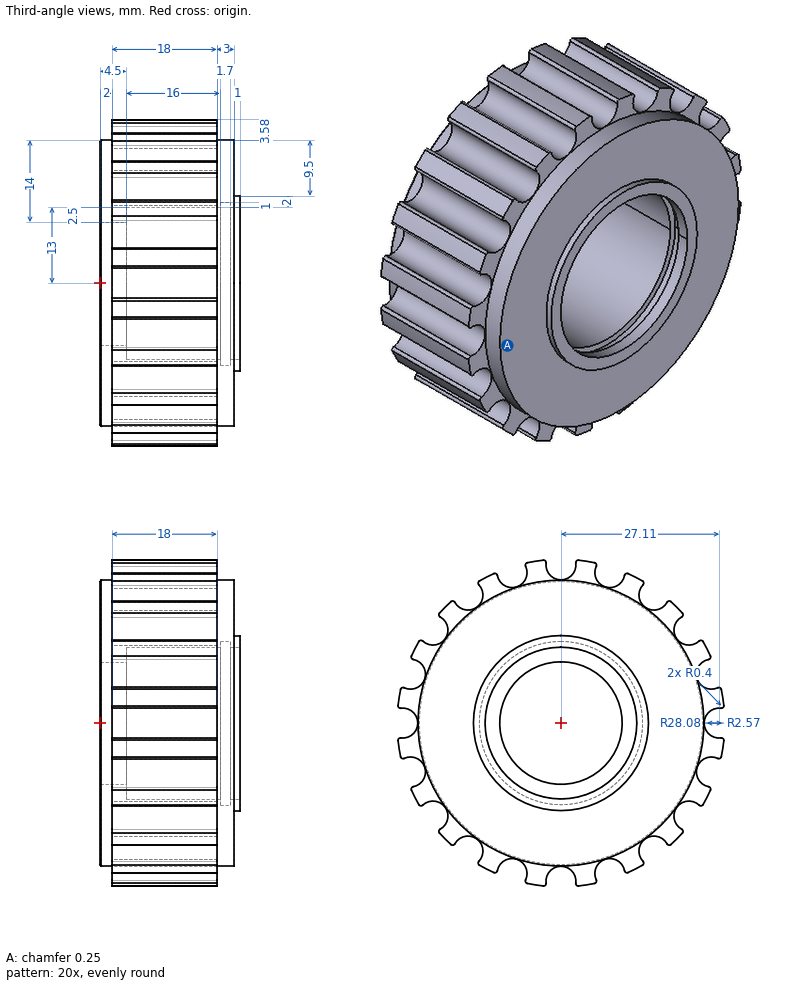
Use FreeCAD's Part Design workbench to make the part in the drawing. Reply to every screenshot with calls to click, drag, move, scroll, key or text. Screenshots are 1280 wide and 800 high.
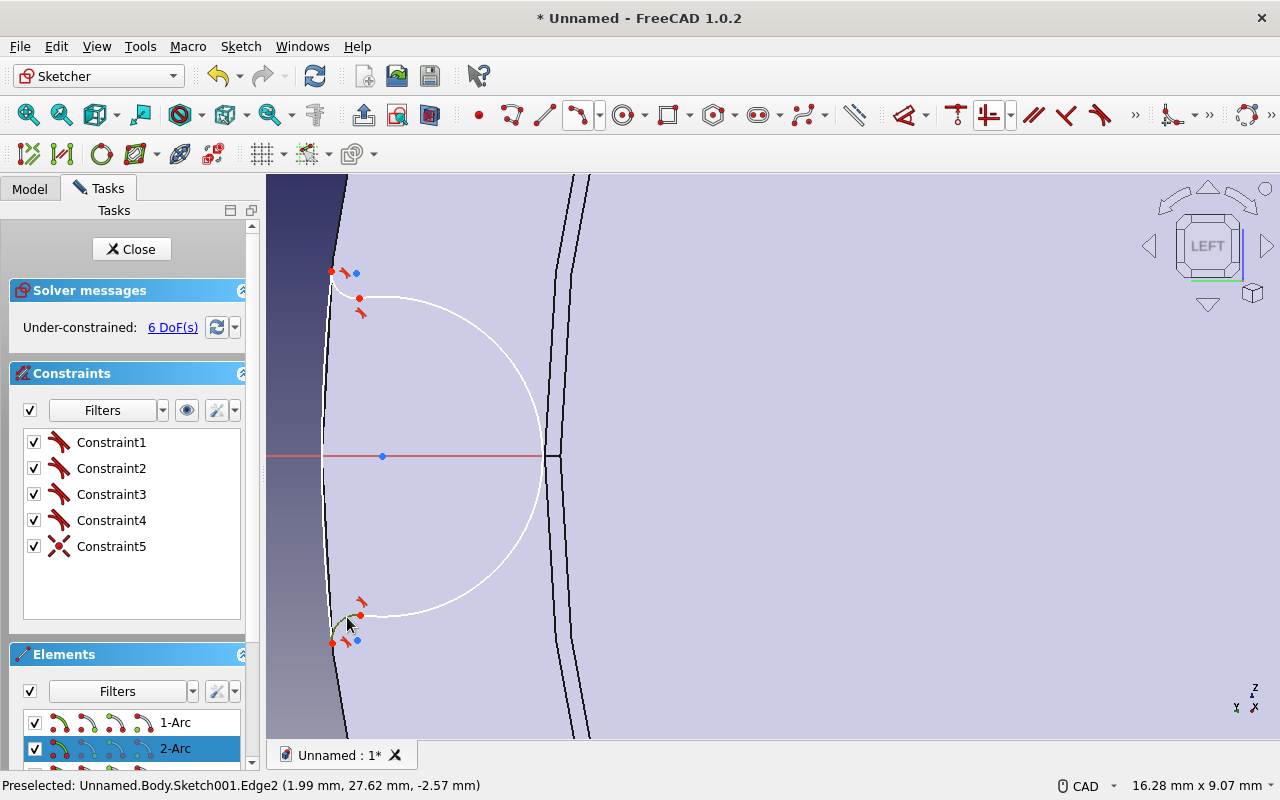
click(347, 296)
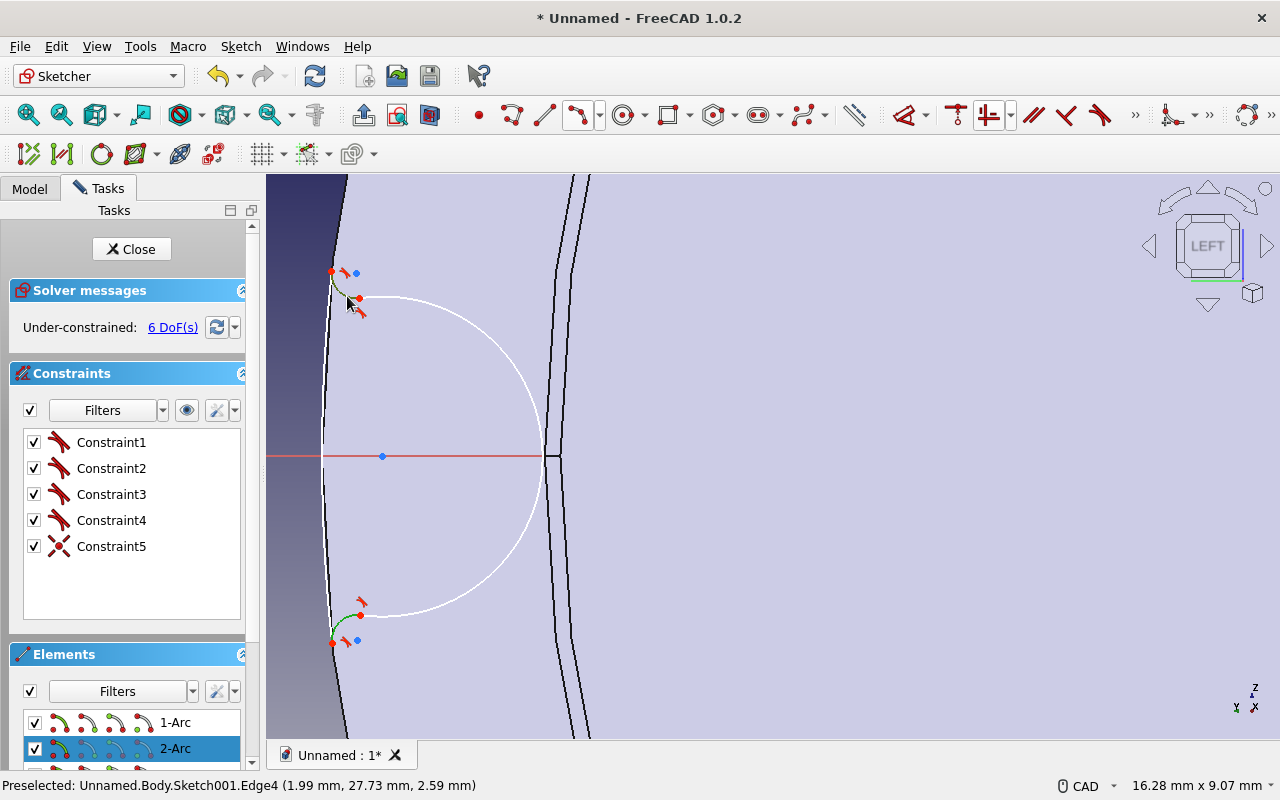
key(e)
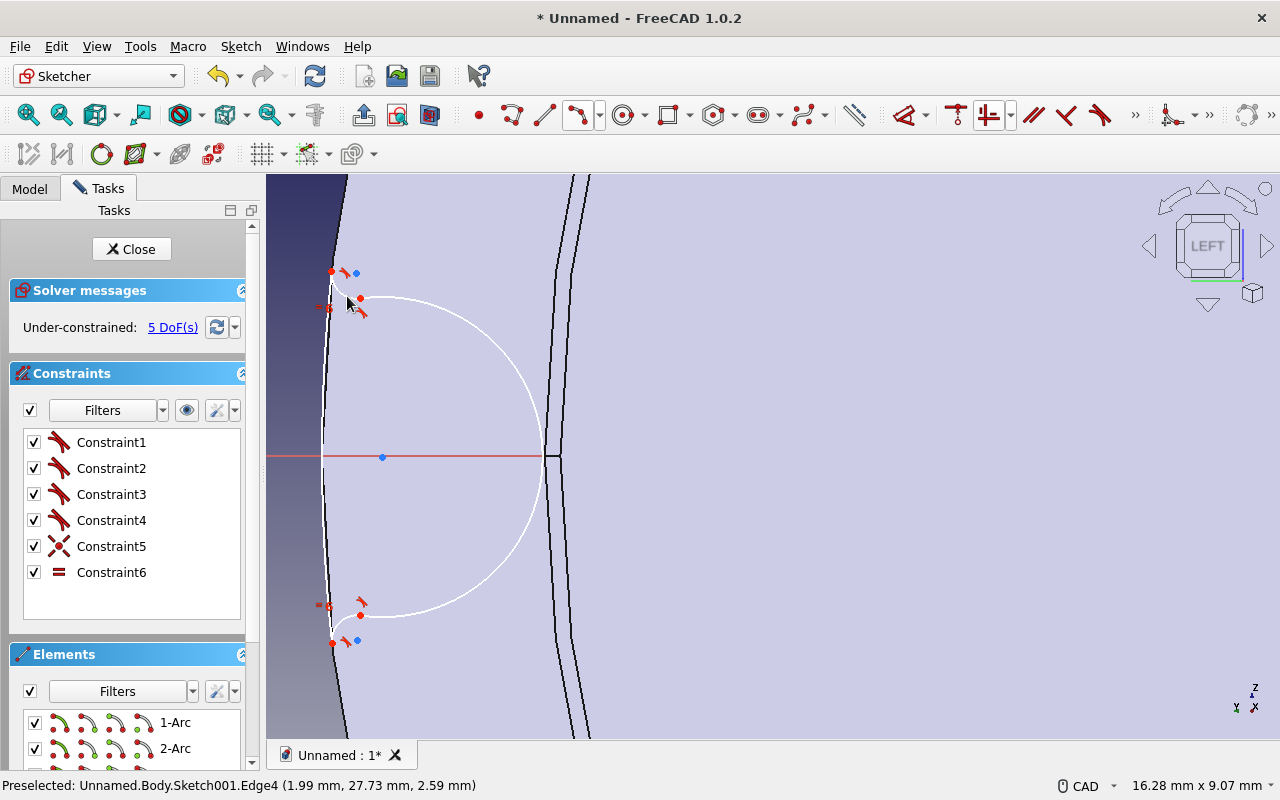
click(383, 457)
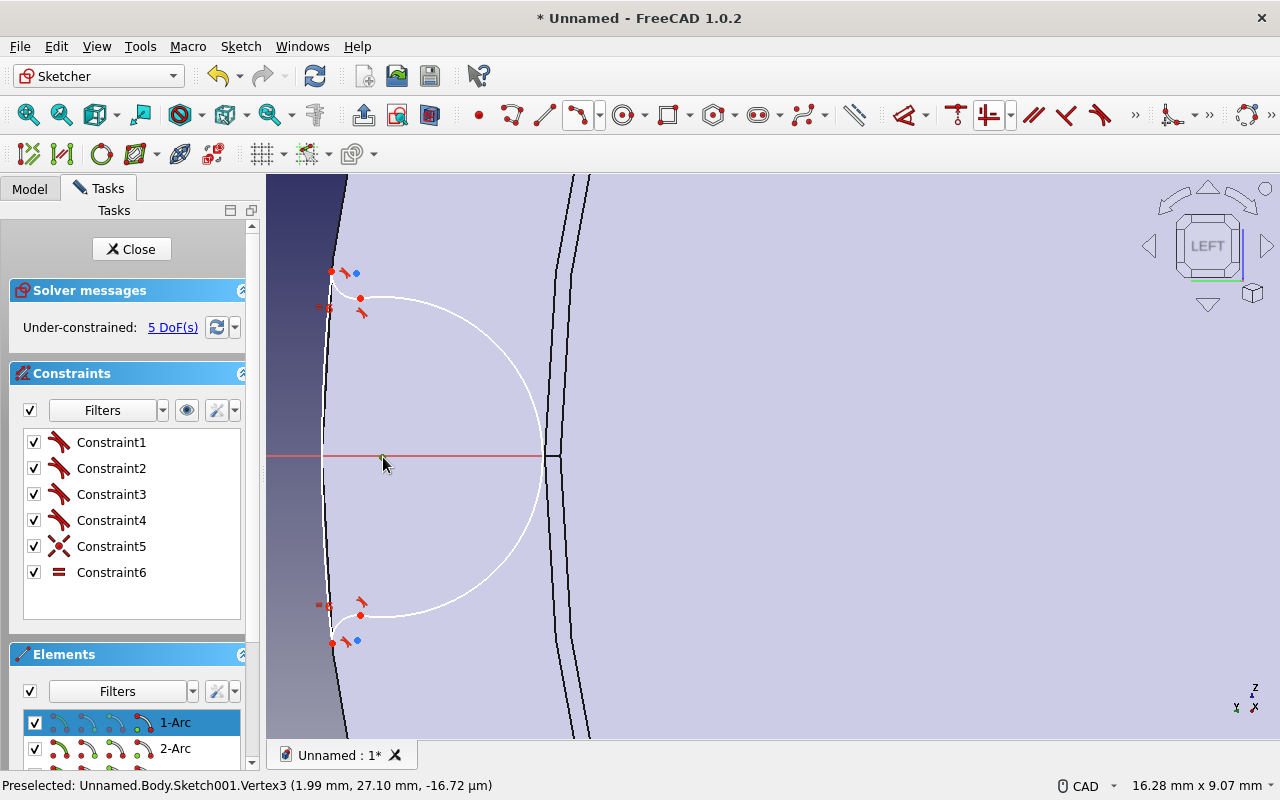
click(353, 456)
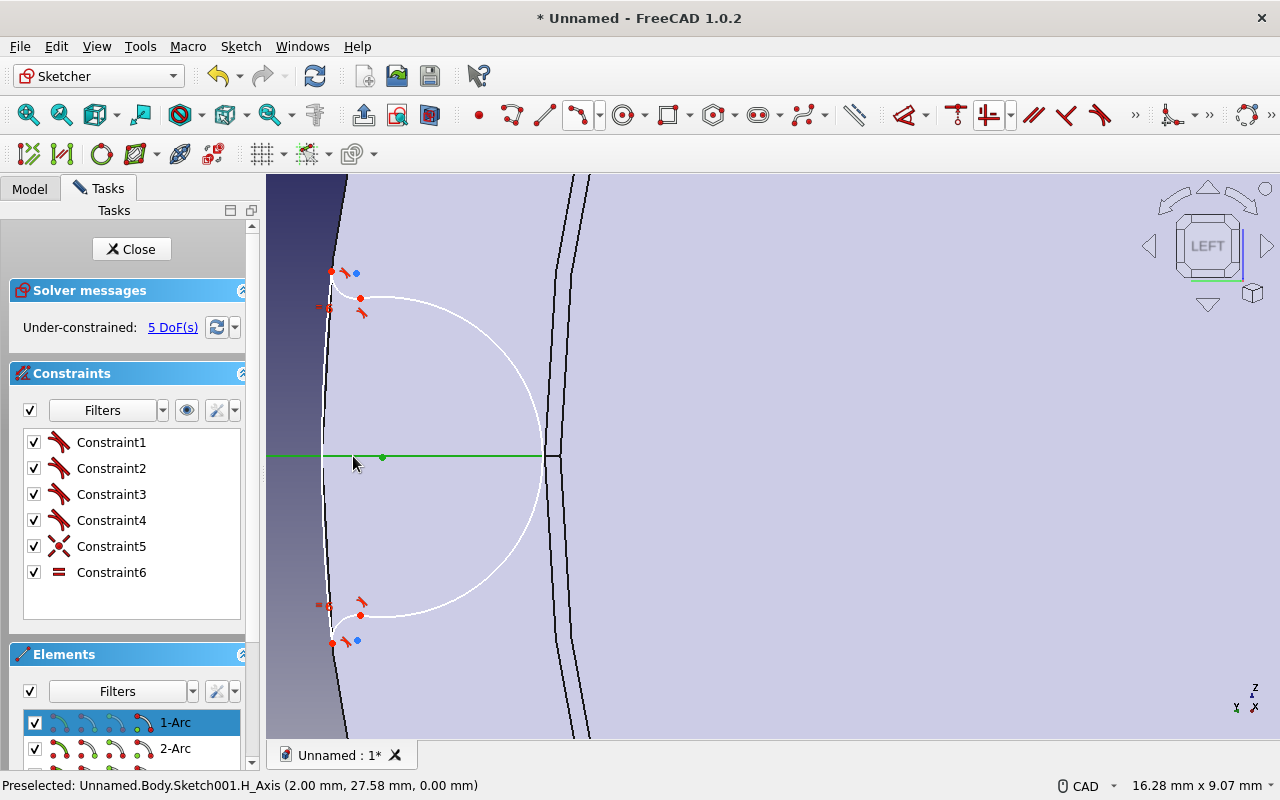
click(956, 116)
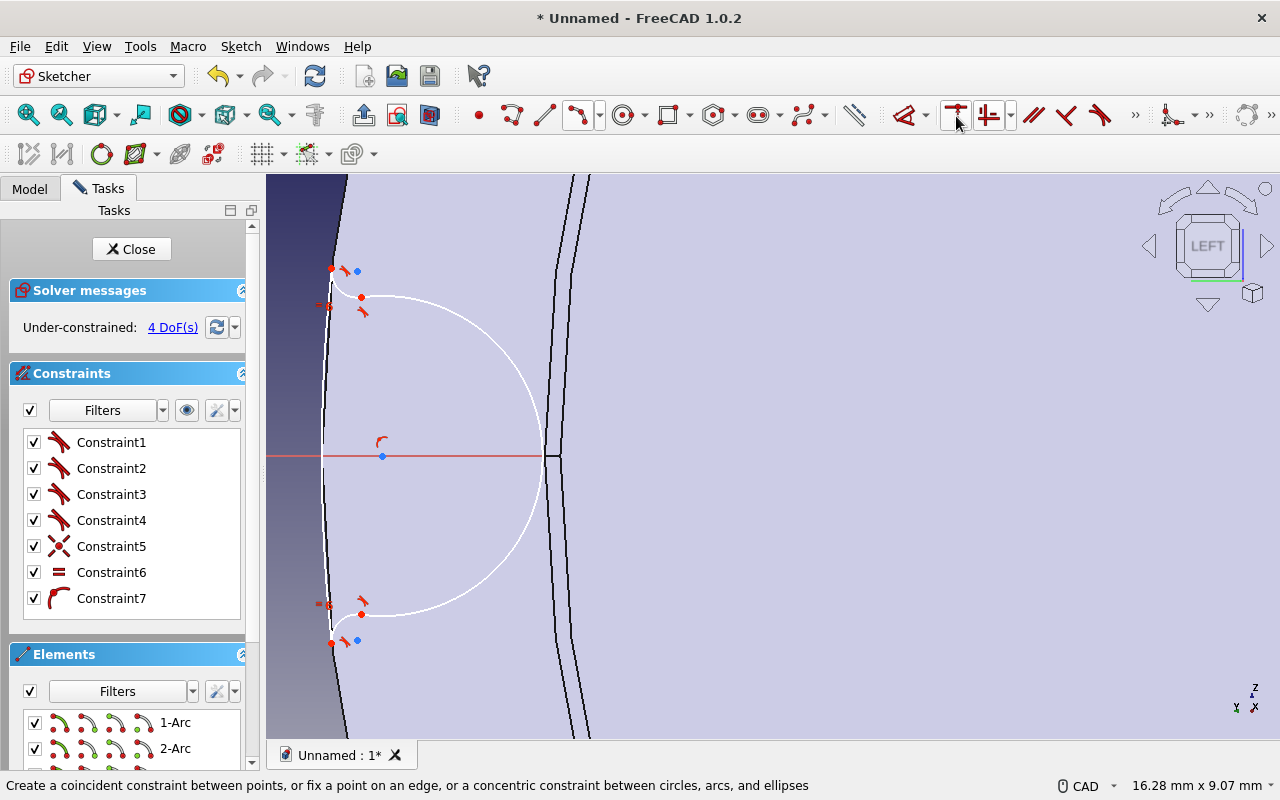
click(904, 116)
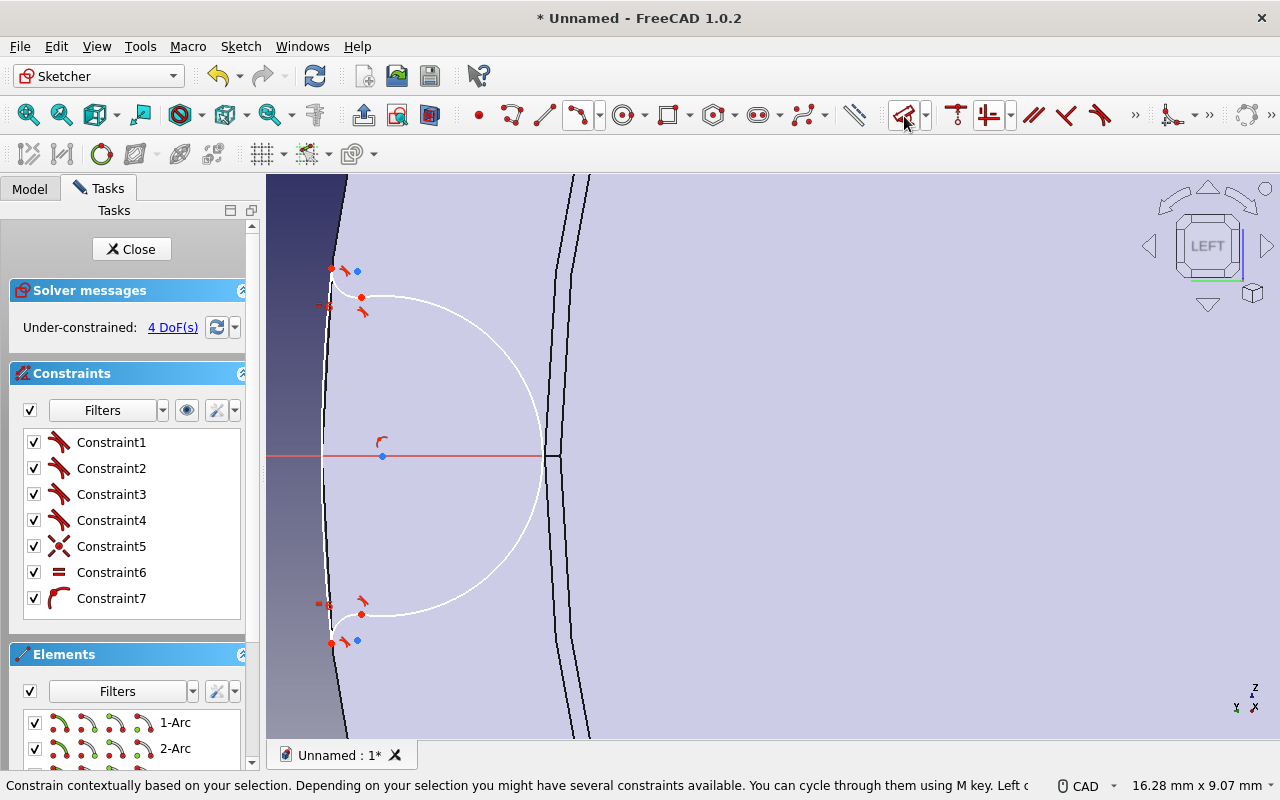
click(507, 557)
click(532, 577)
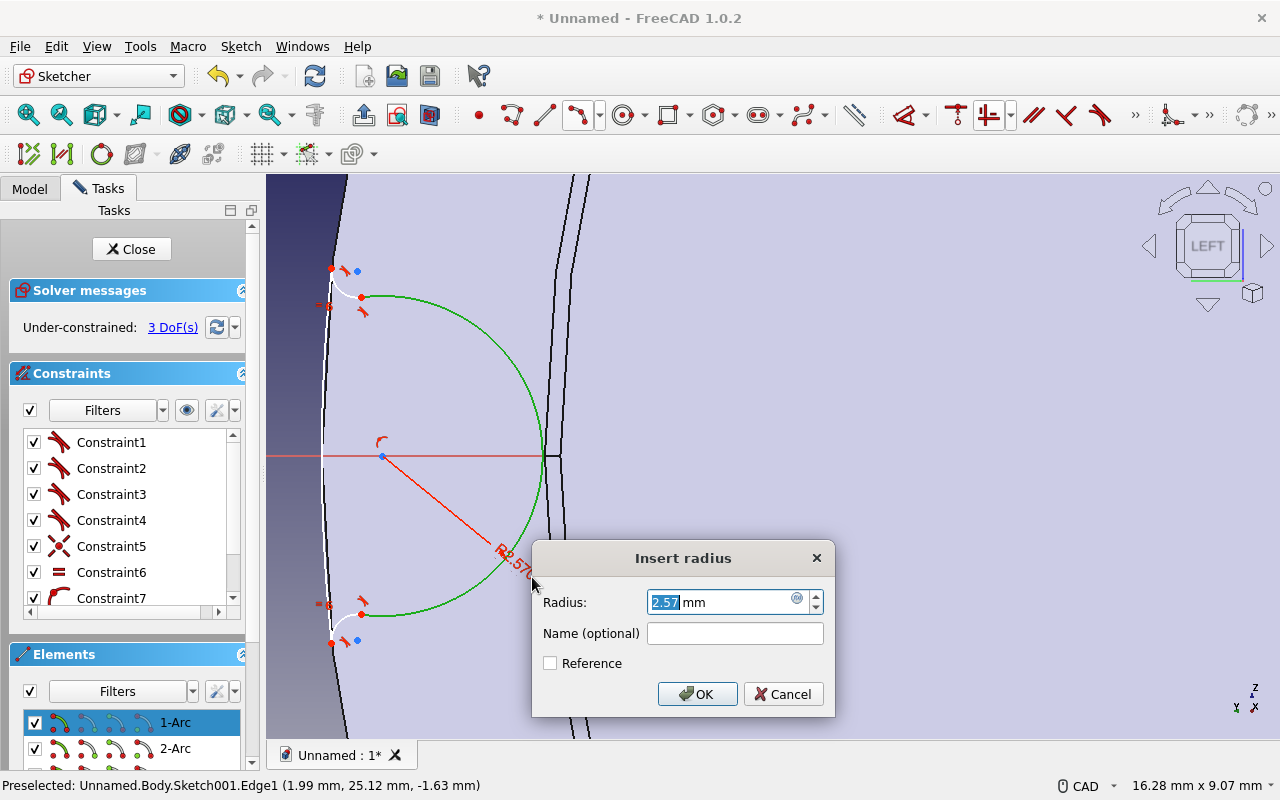
text(2.57)
key(Return)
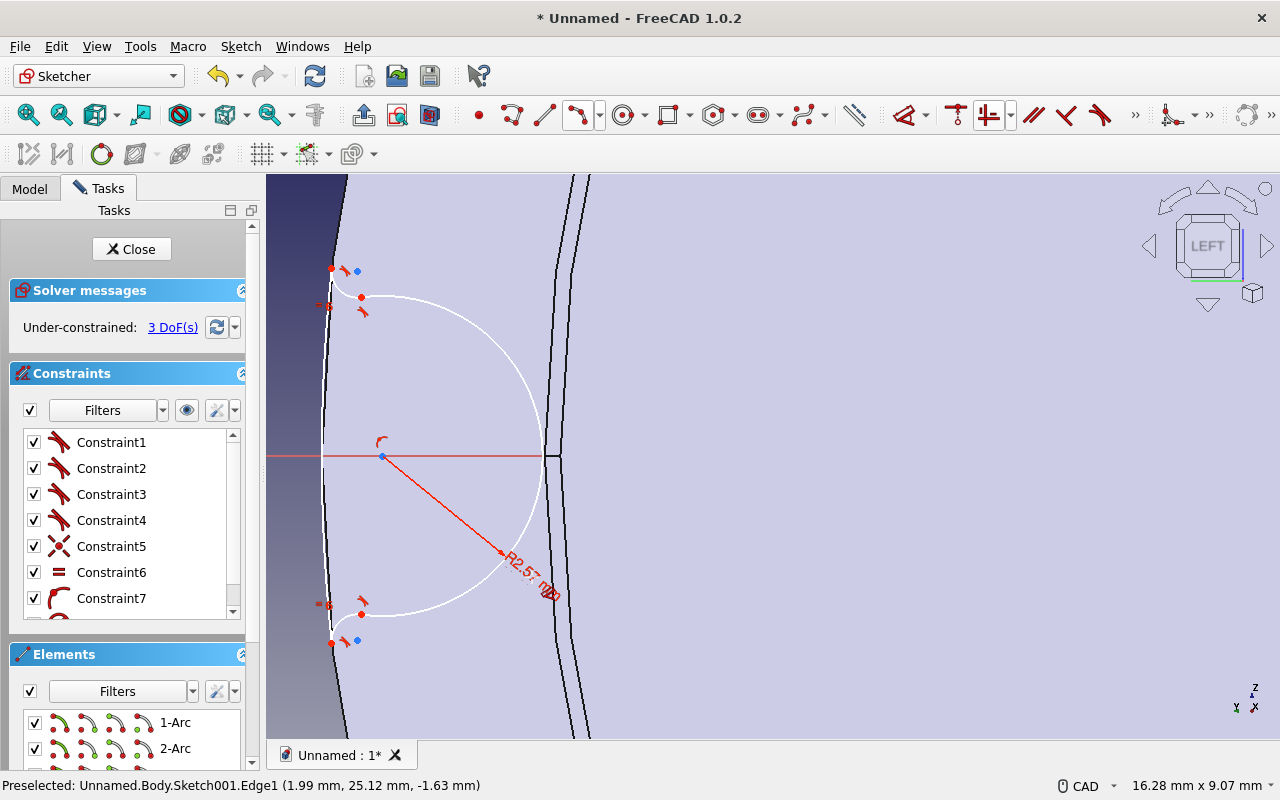
scroll(347, 617, up, 3)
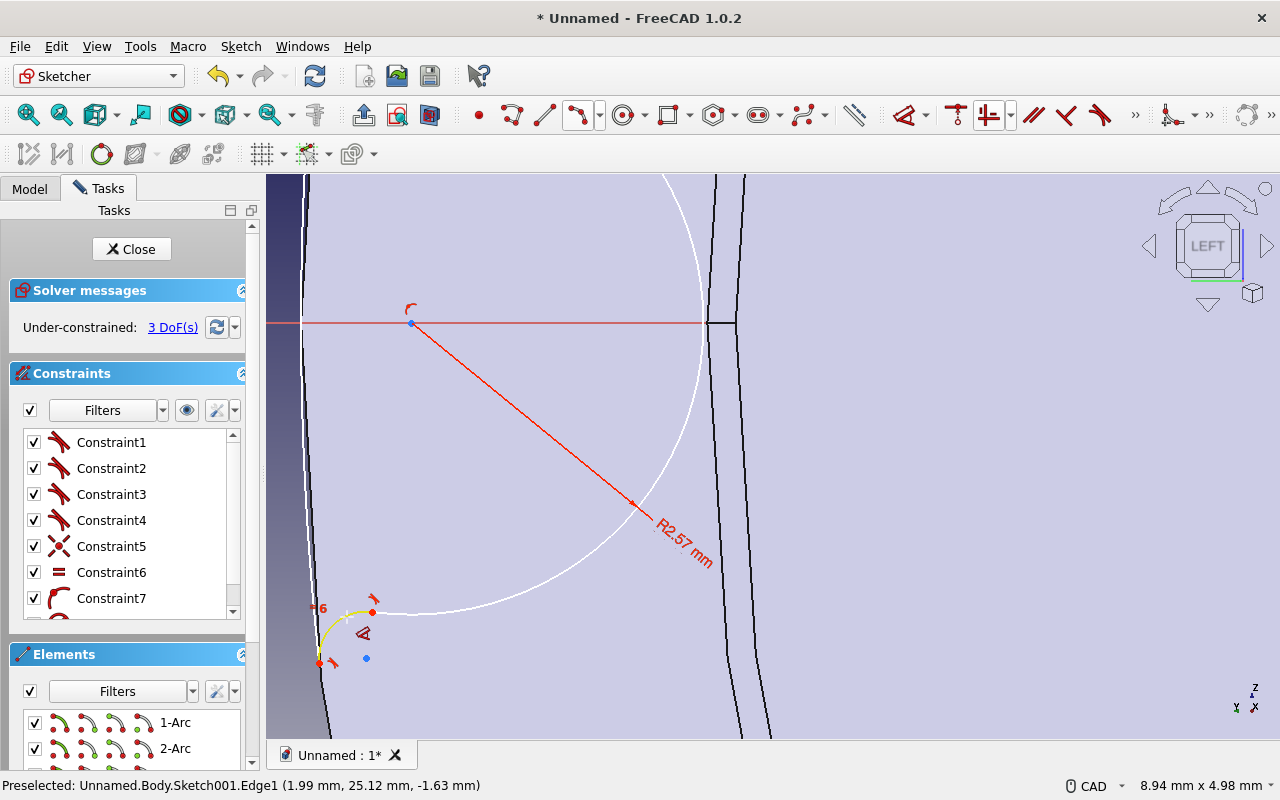
click(348, 616)
click(335, 587)